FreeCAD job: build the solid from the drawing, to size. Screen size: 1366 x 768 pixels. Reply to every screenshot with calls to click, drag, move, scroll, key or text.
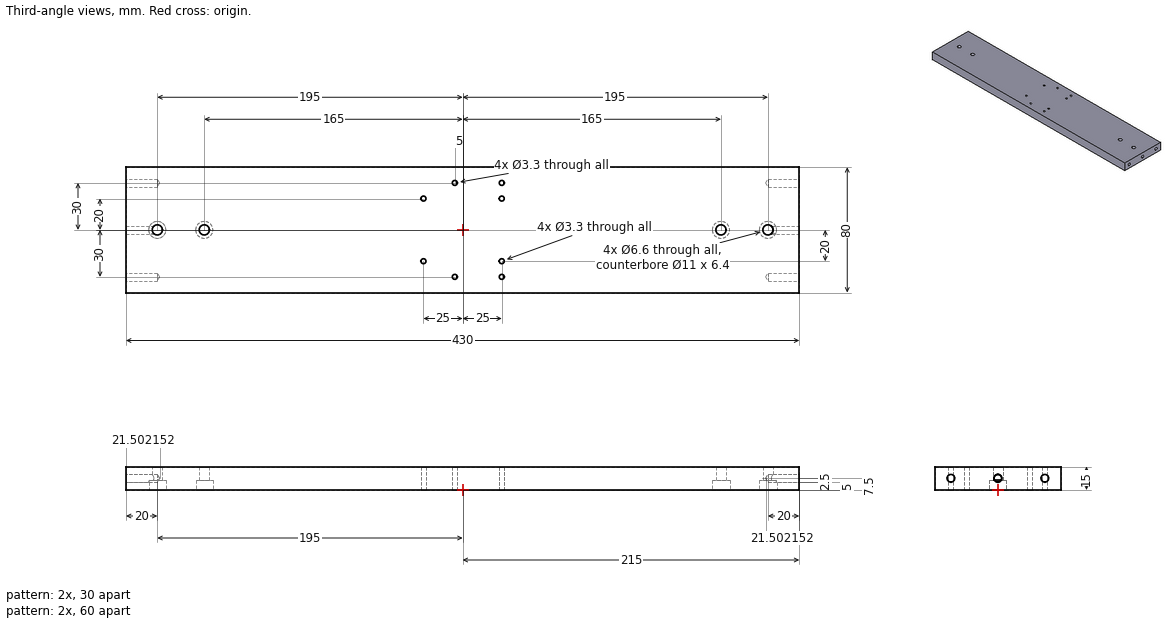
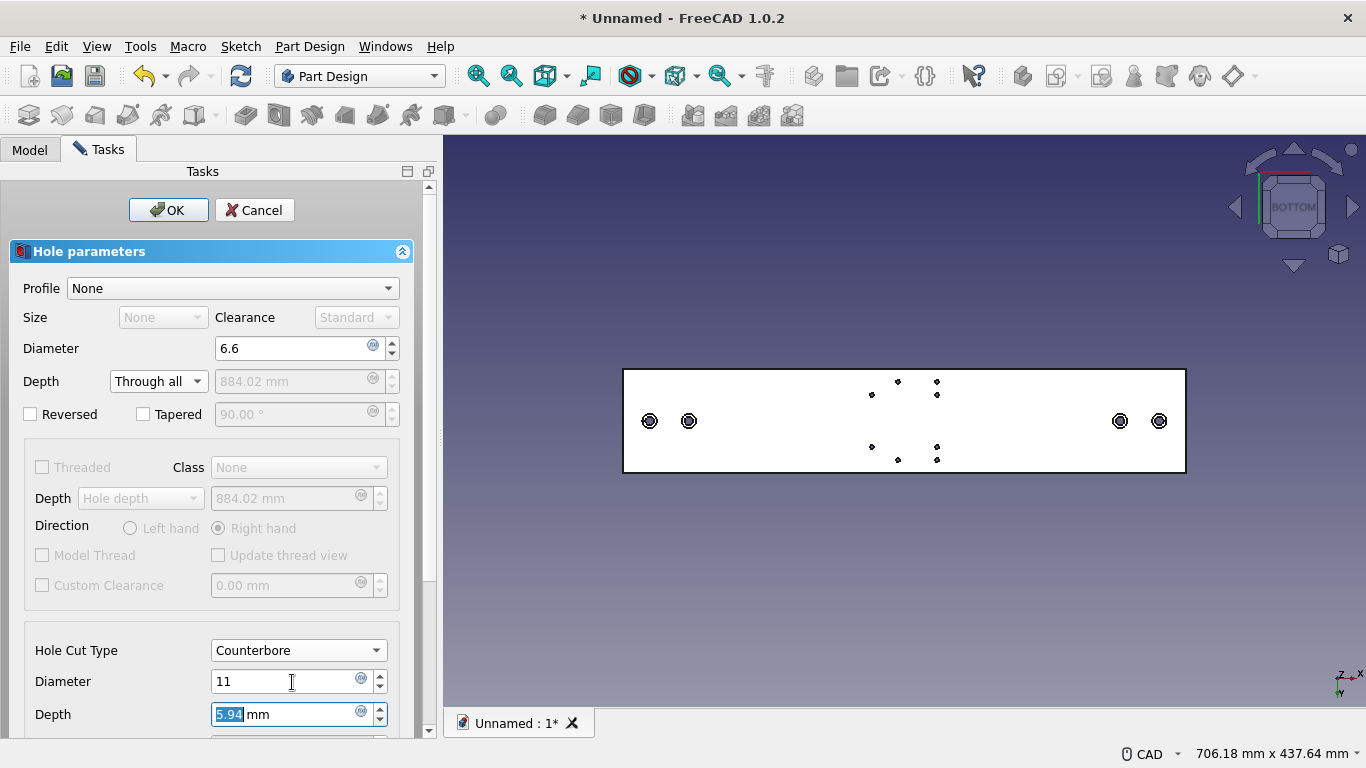
text(6.4)
key(Tab)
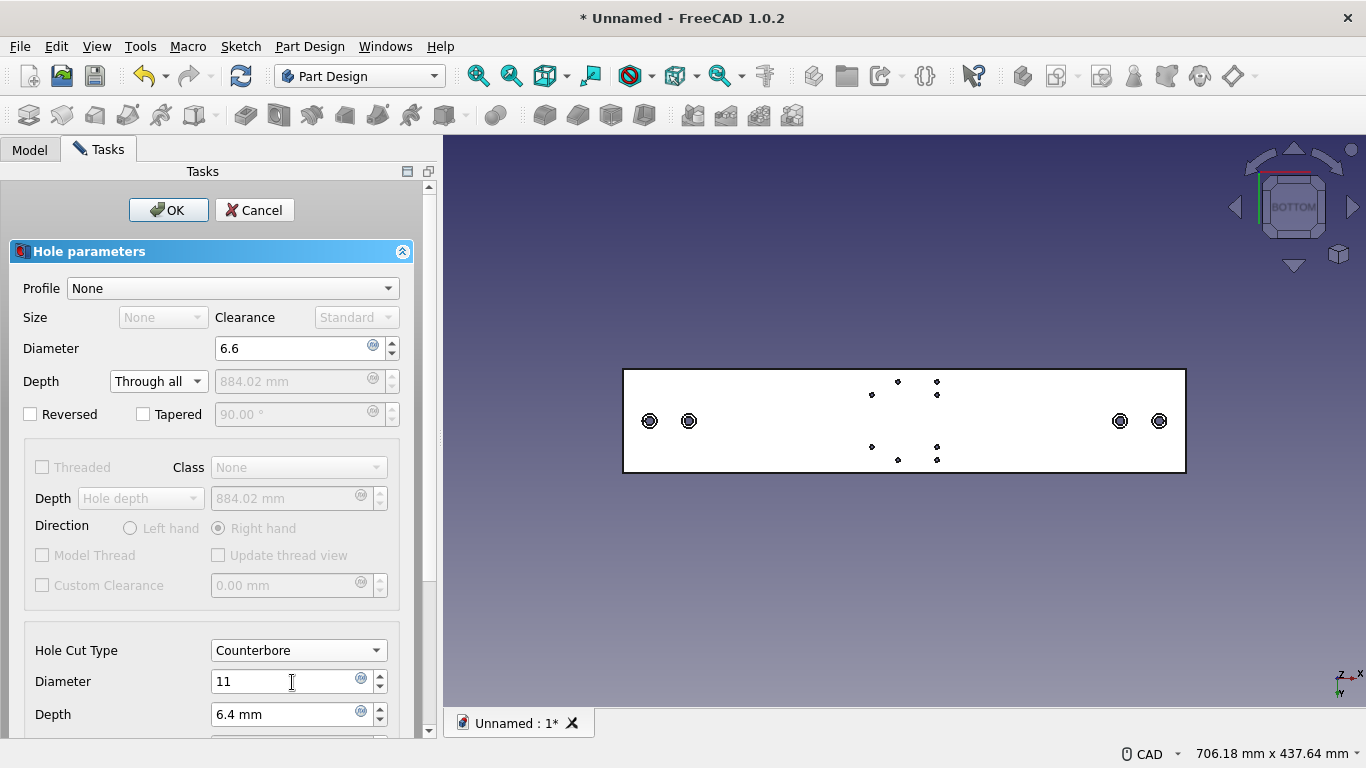
click(169, 210)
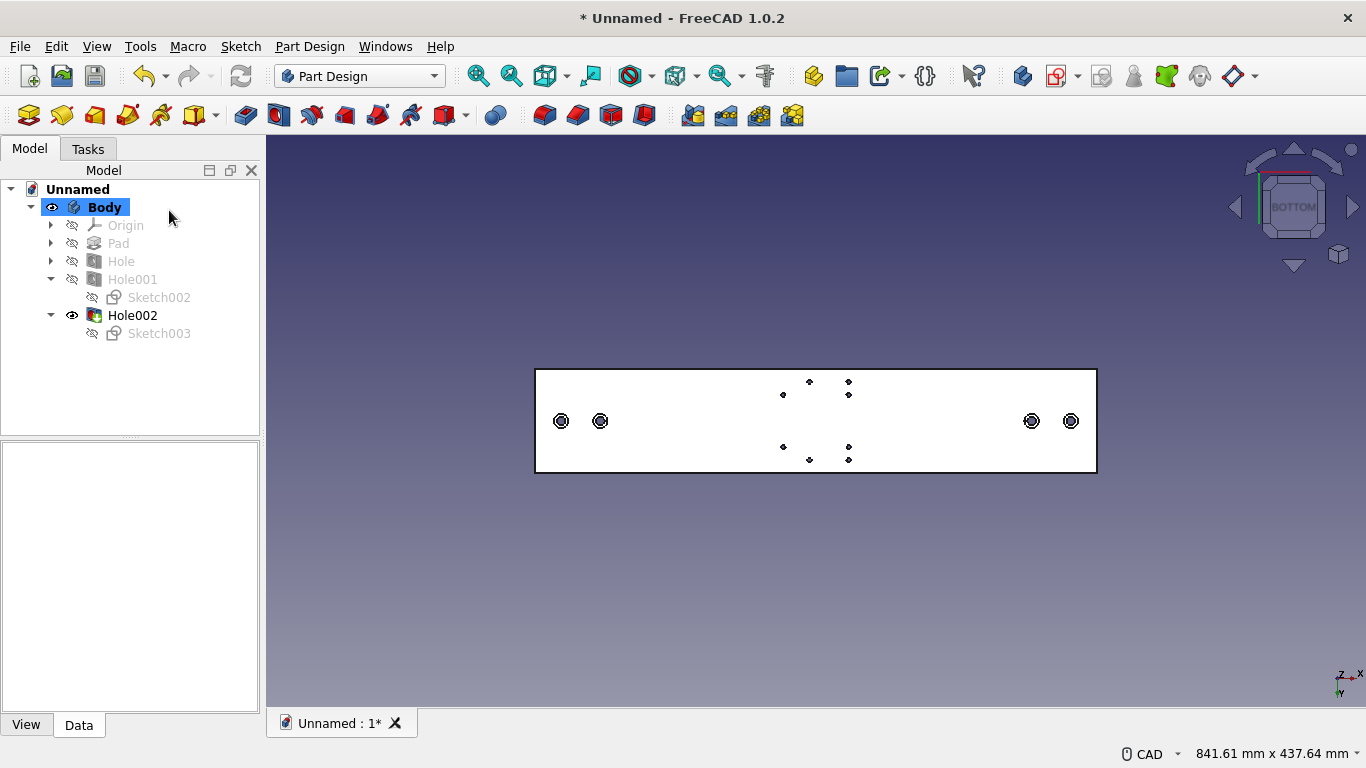
click(51, 225)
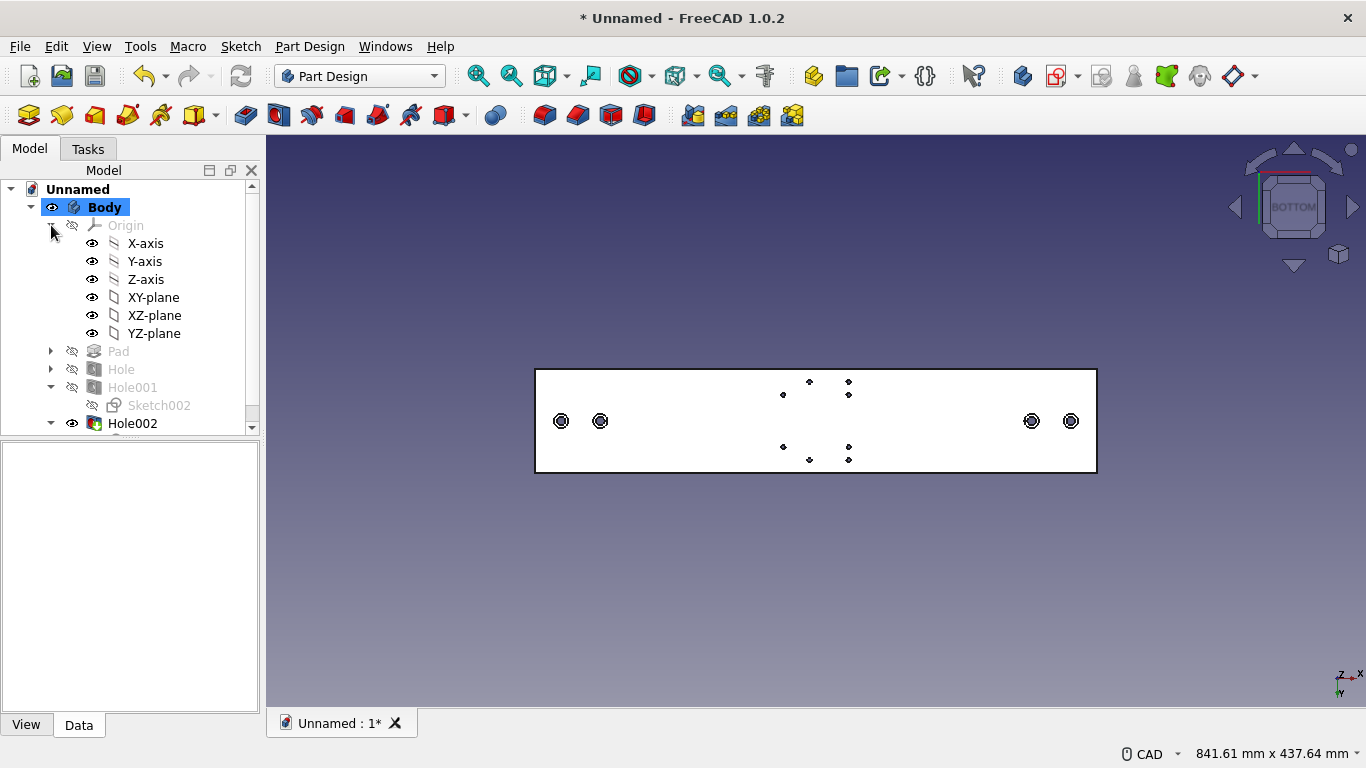
click(137, 315)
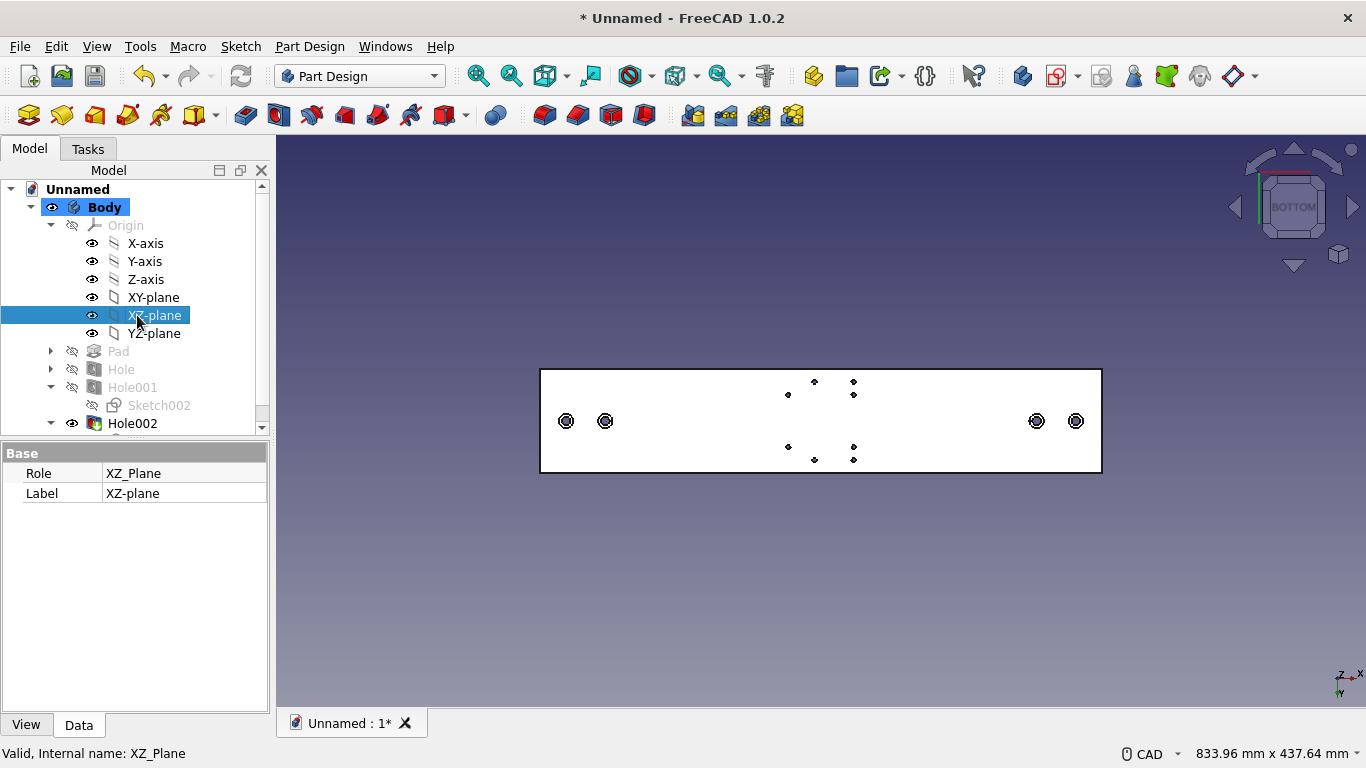
click(1232, 76)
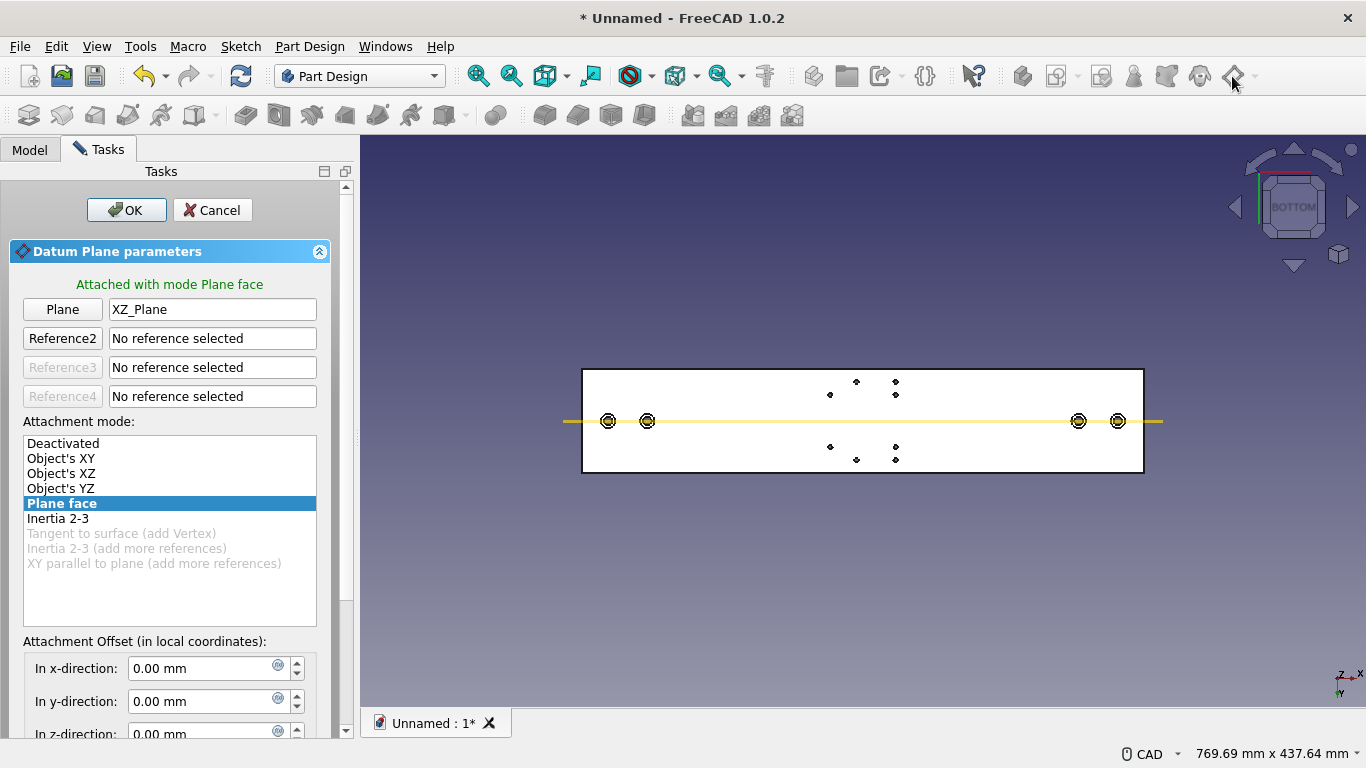
scroll(346, 460, down, 2)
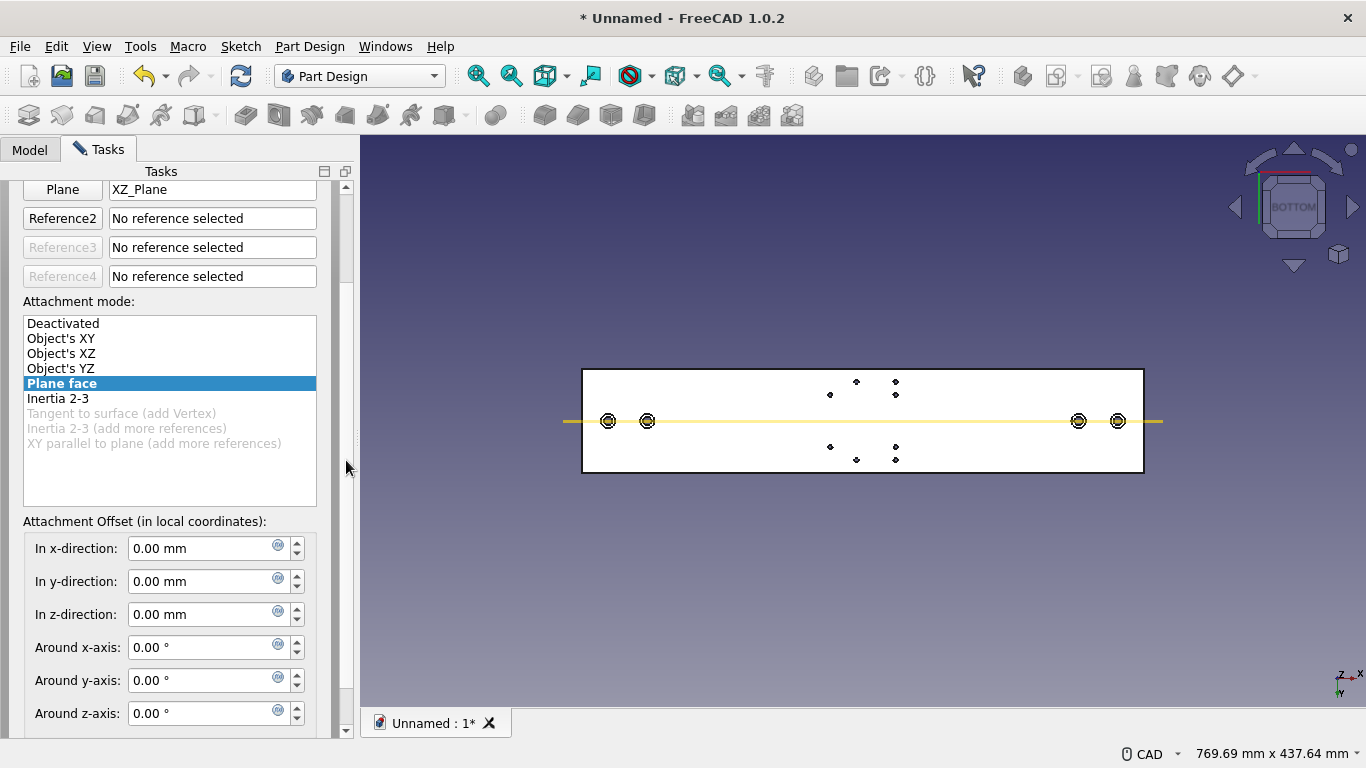
triple_click(210, 614)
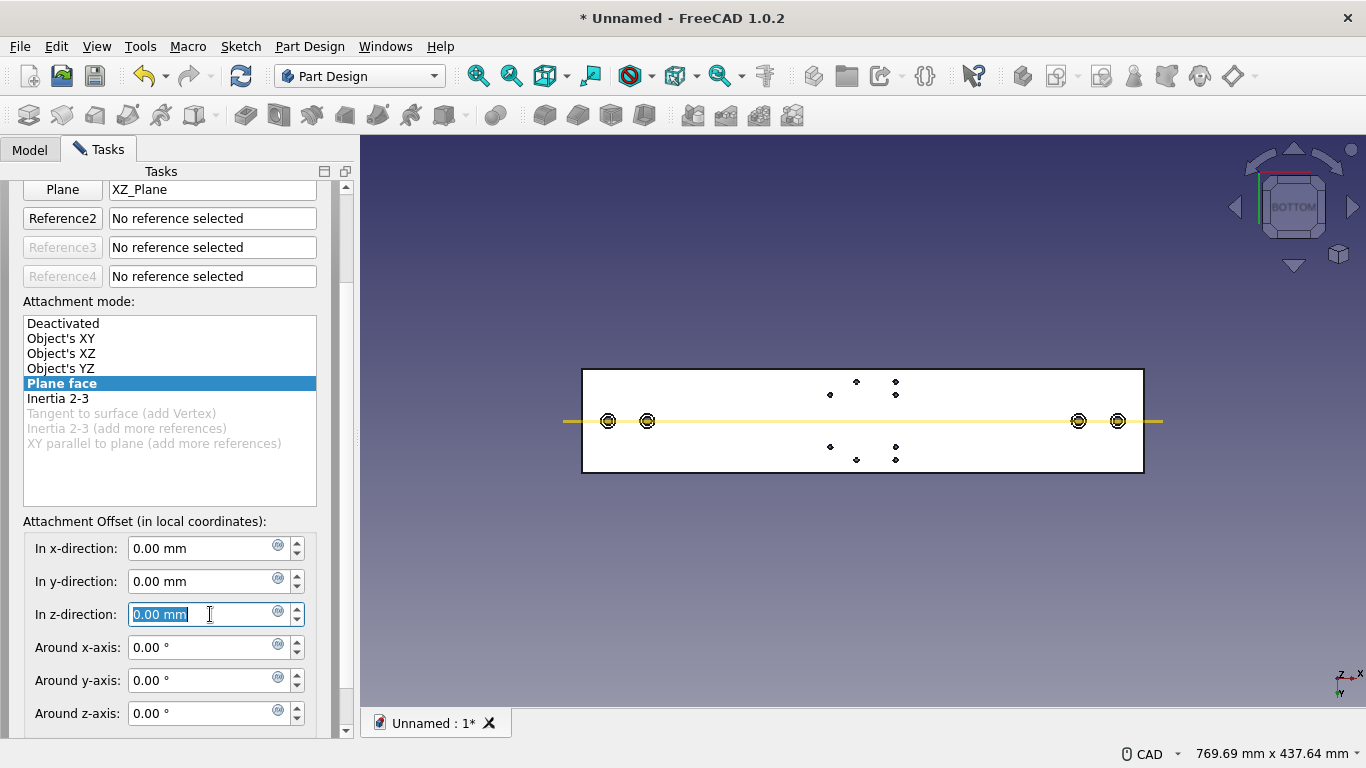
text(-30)
key(Tab)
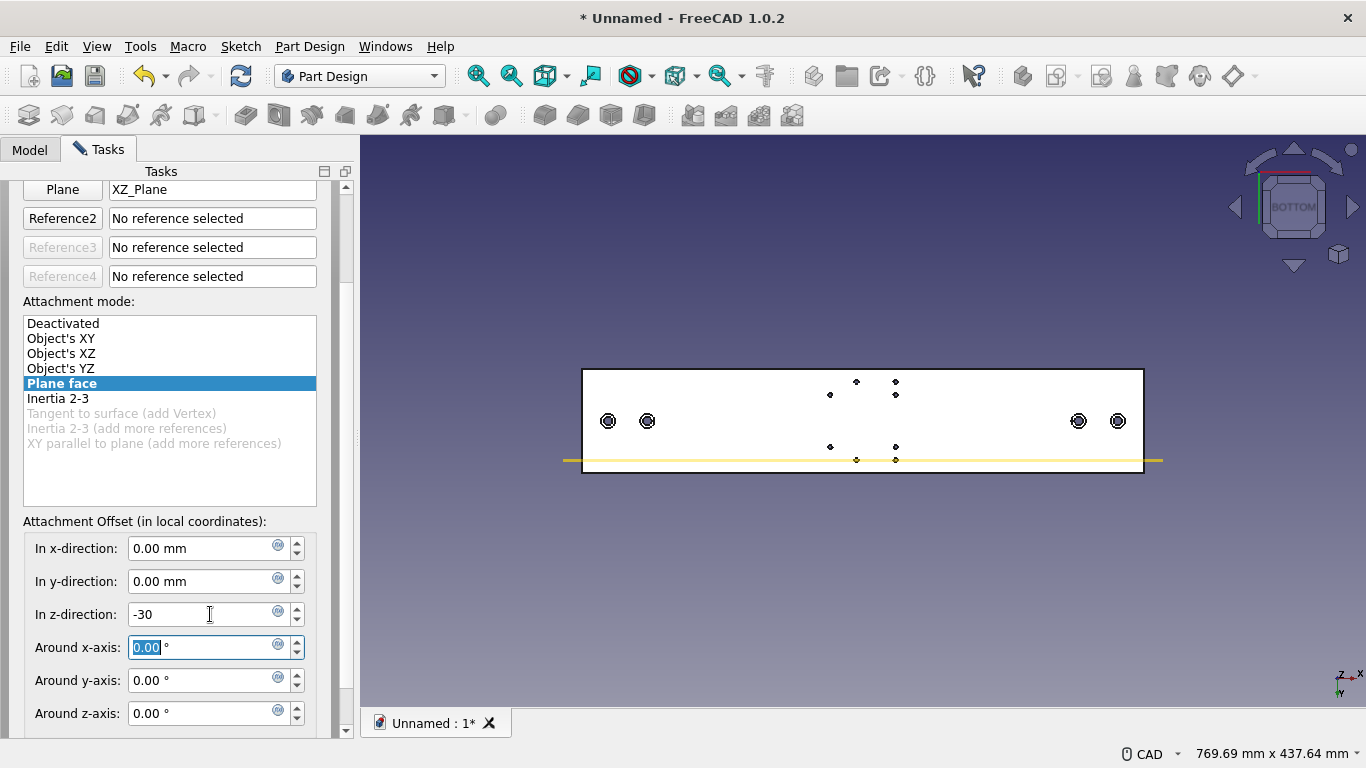
scroll(346, 460, up, 3)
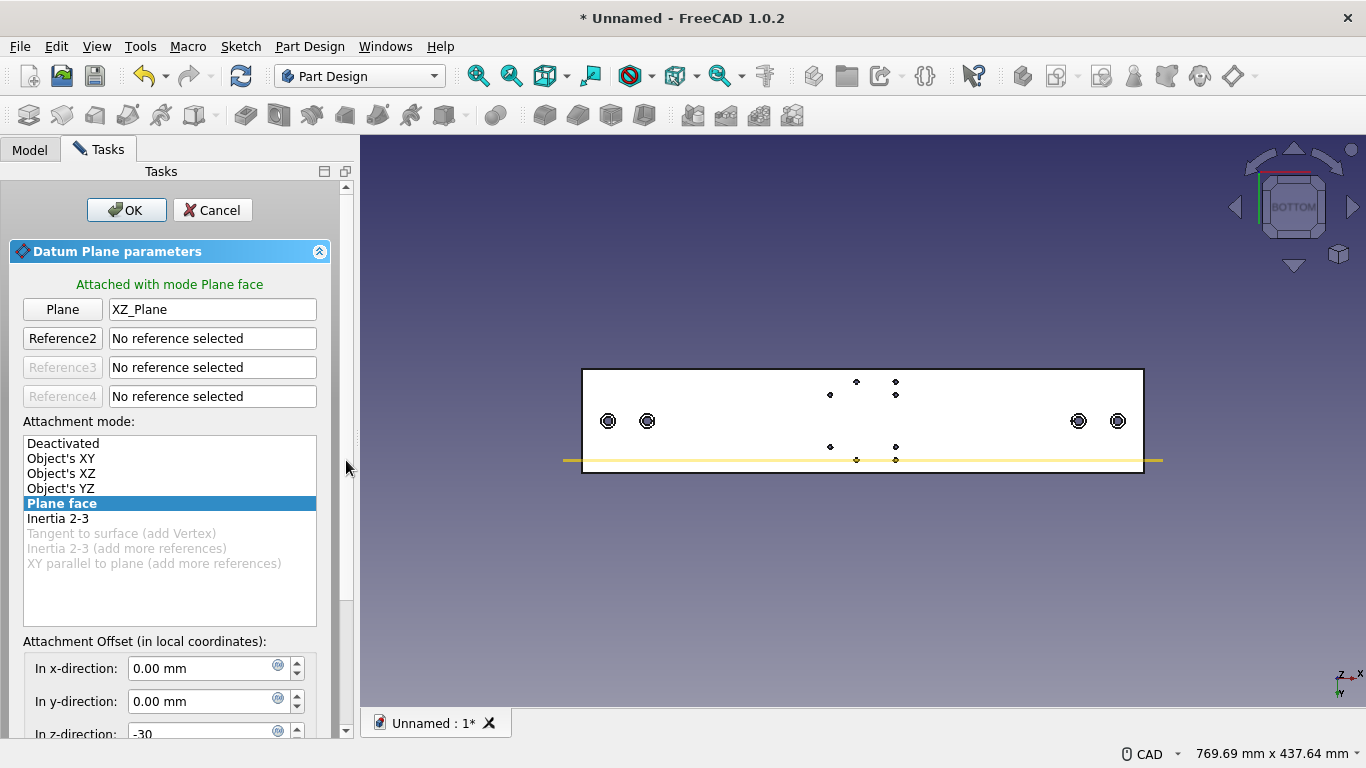
click(127, 210)